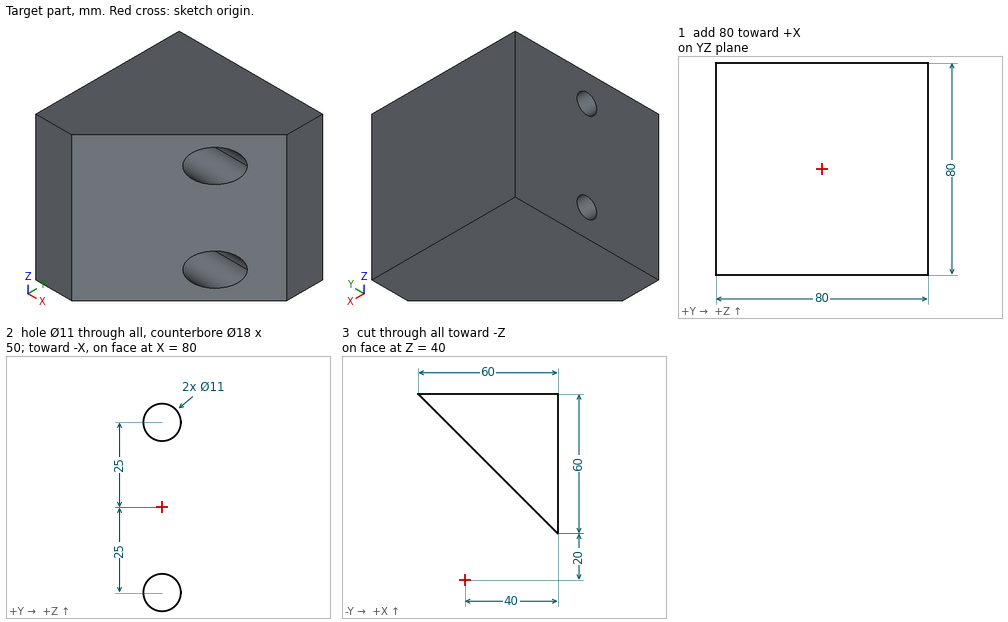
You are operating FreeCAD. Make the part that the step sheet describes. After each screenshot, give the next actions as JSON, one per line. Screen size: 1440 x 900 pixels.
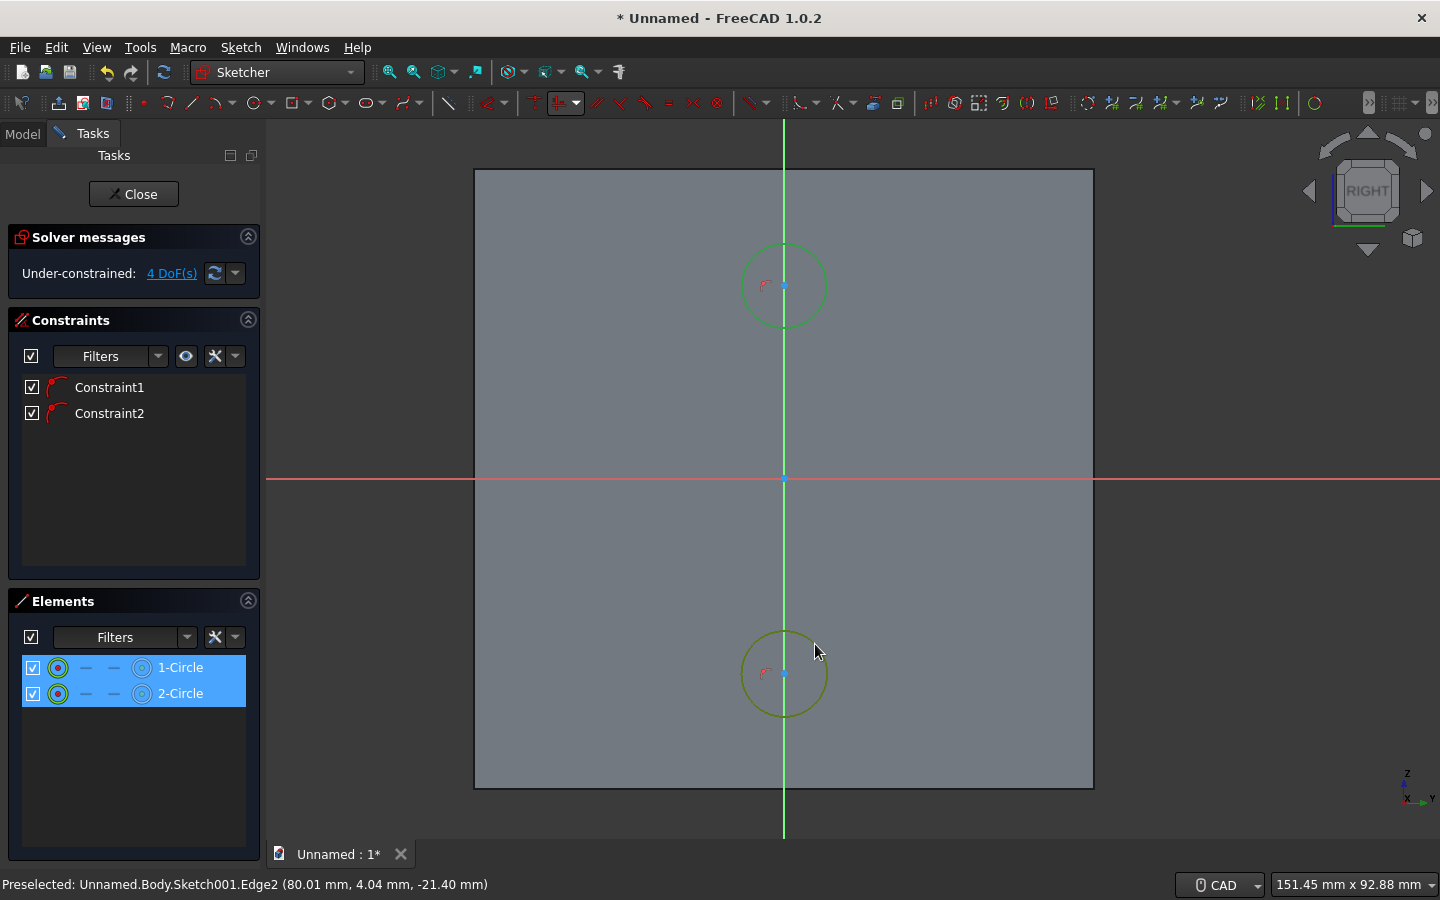
{"action": "key", "text": "e"}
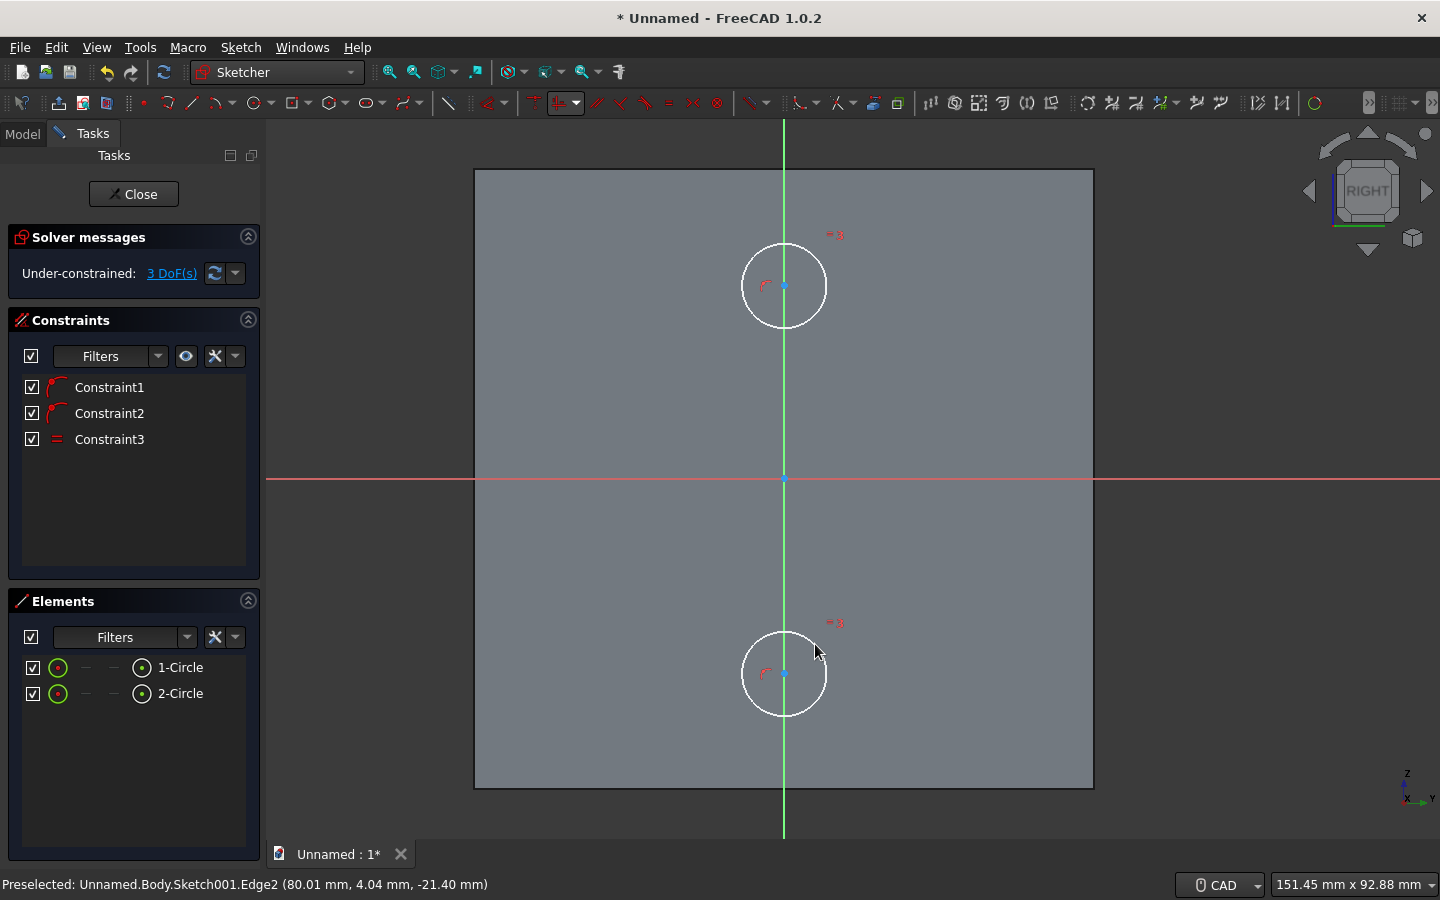
{"action": "key", "text": "d"}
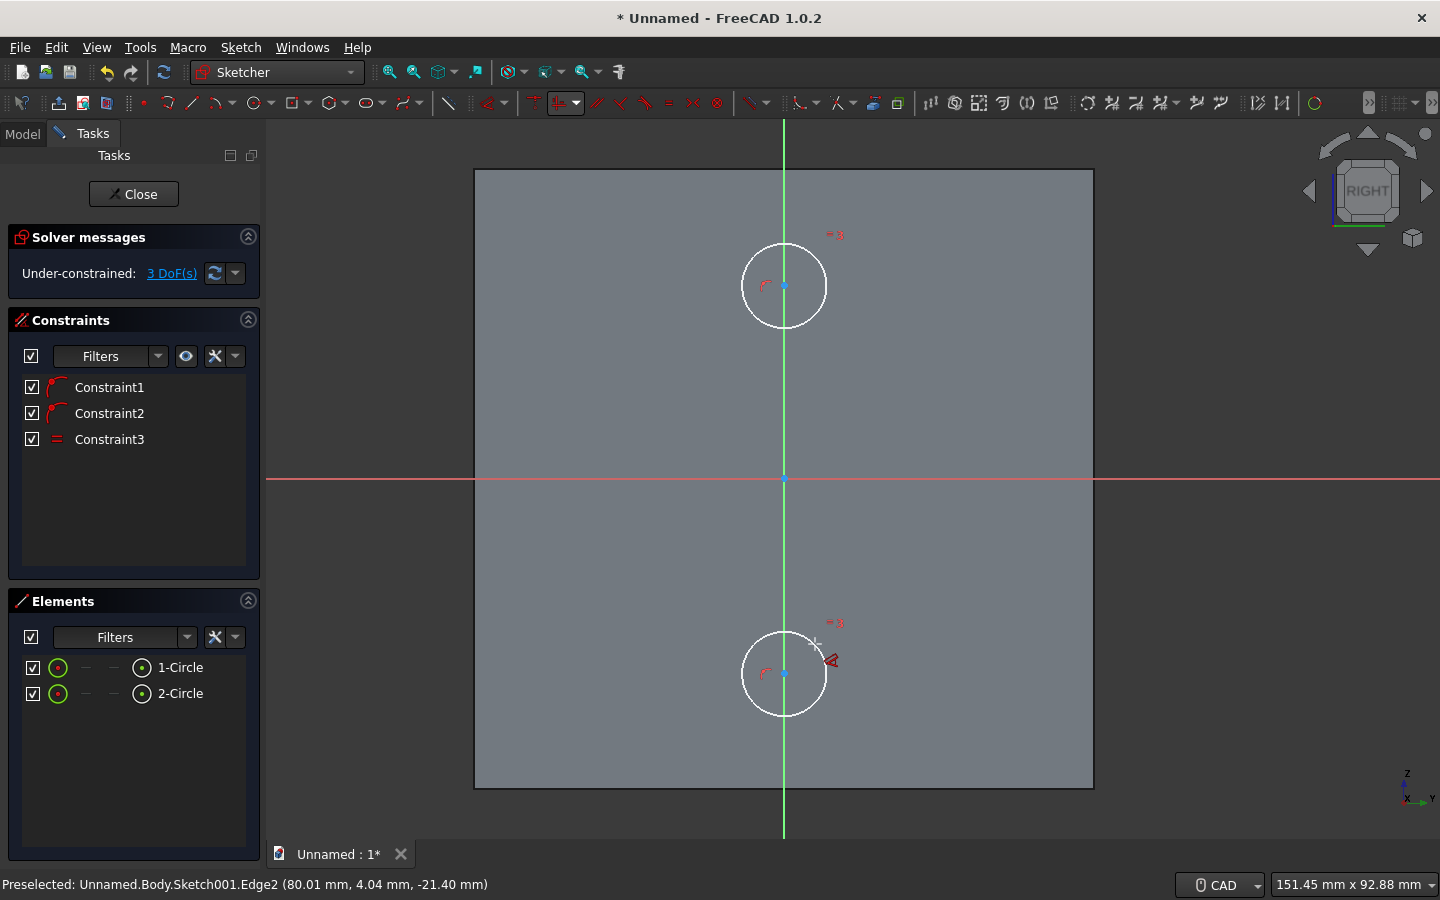
{"action": "left_click", "coordinate": [814, 256]}
{"action": "left_click", "coordinate": [837, 233]}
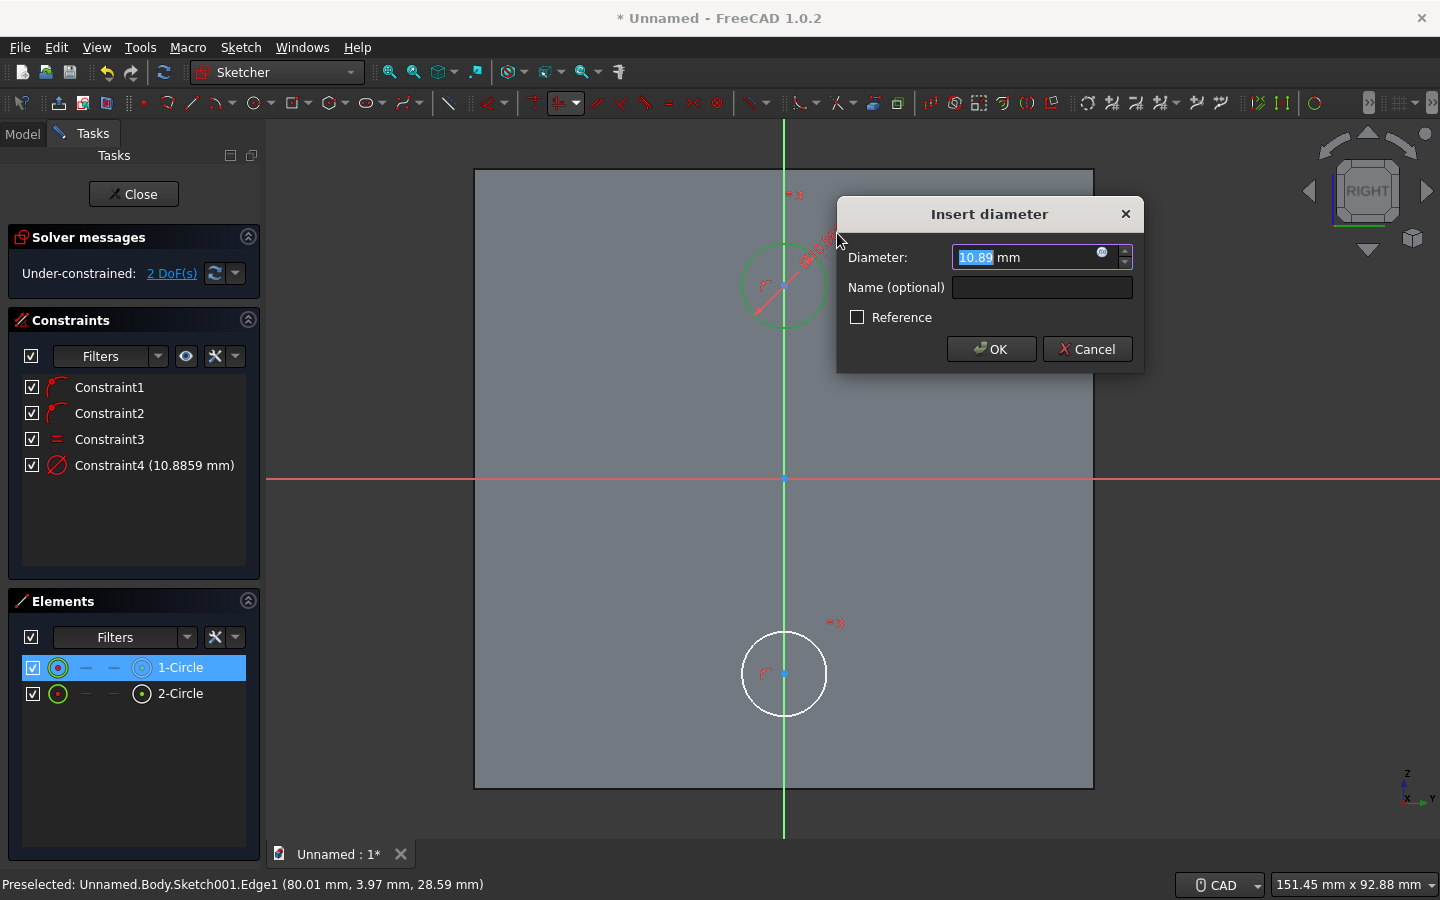
{"action": "type", "text": "11"}
{"action": "key", "text": "Return"}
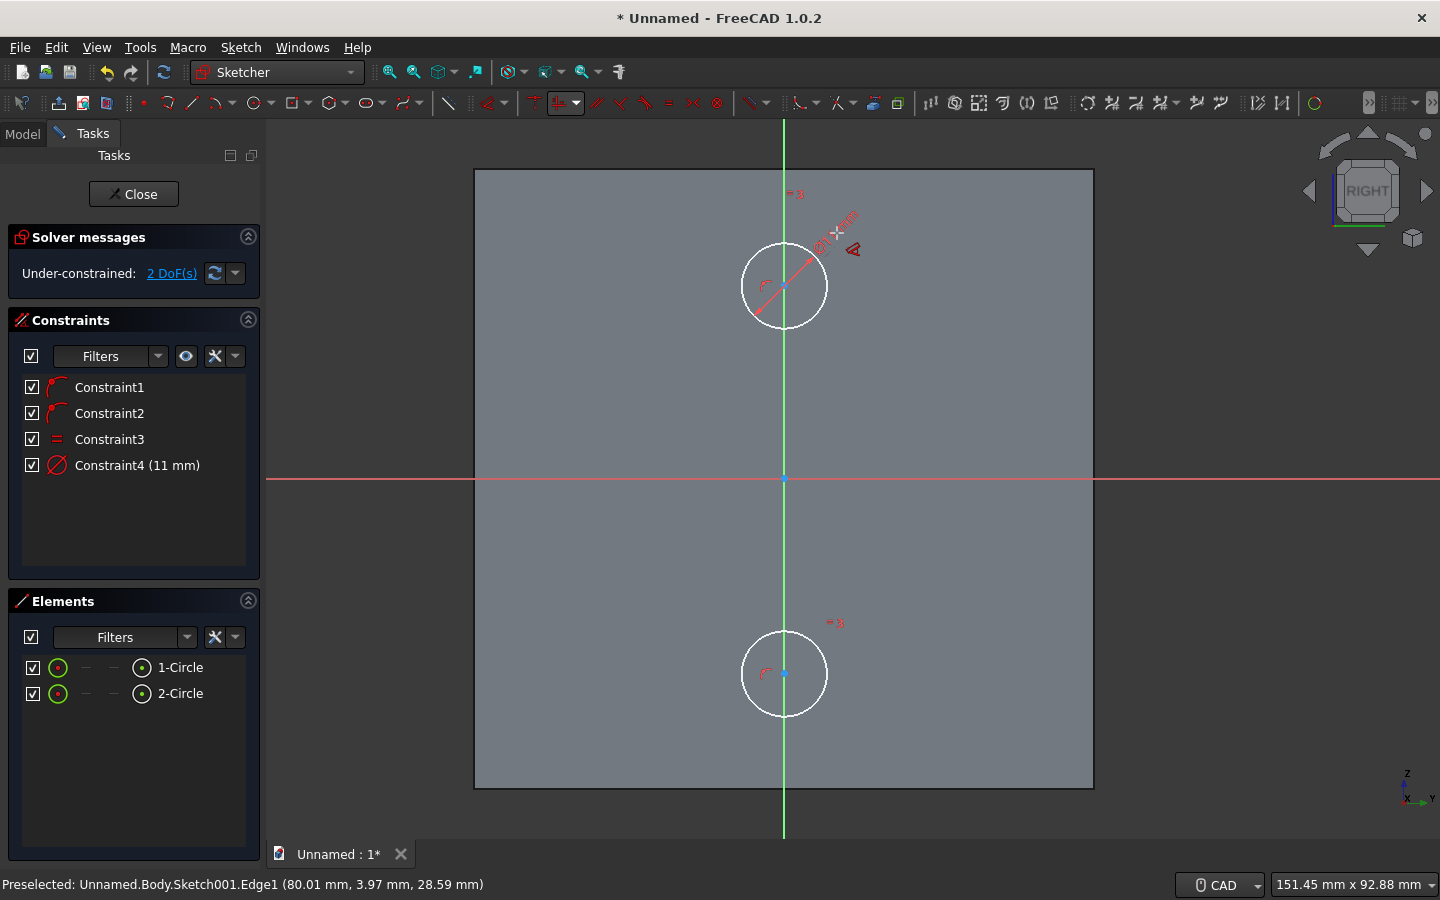
{"action": "left_click", "coordinate": [784, 286]}
{"action": "left_click", "coordinate": [818, 382]}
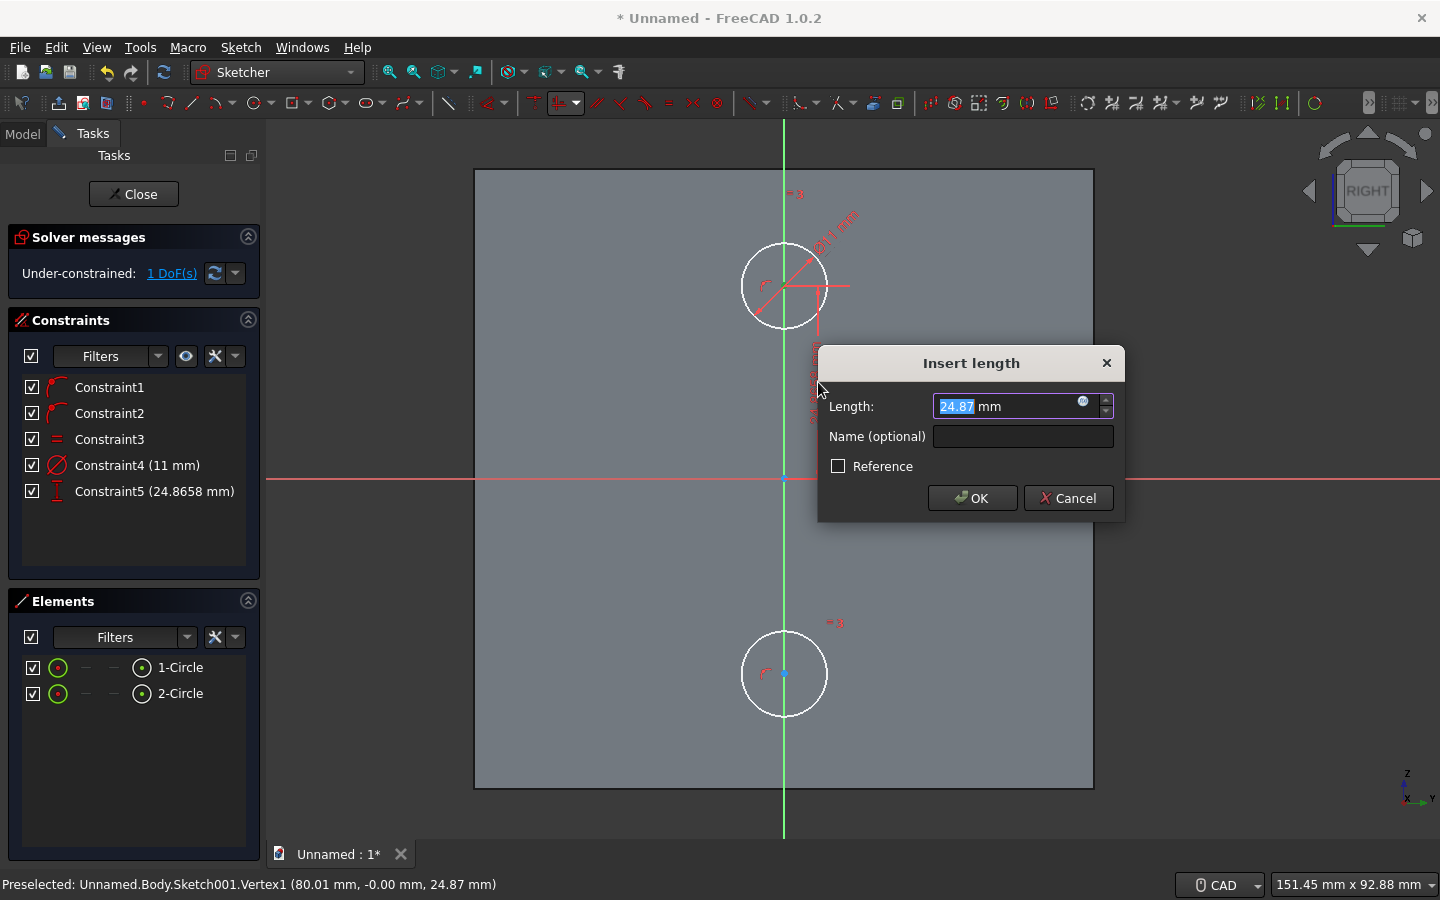
{"action": "type", "text": "25"}
{"action": "key", "text": "Return"}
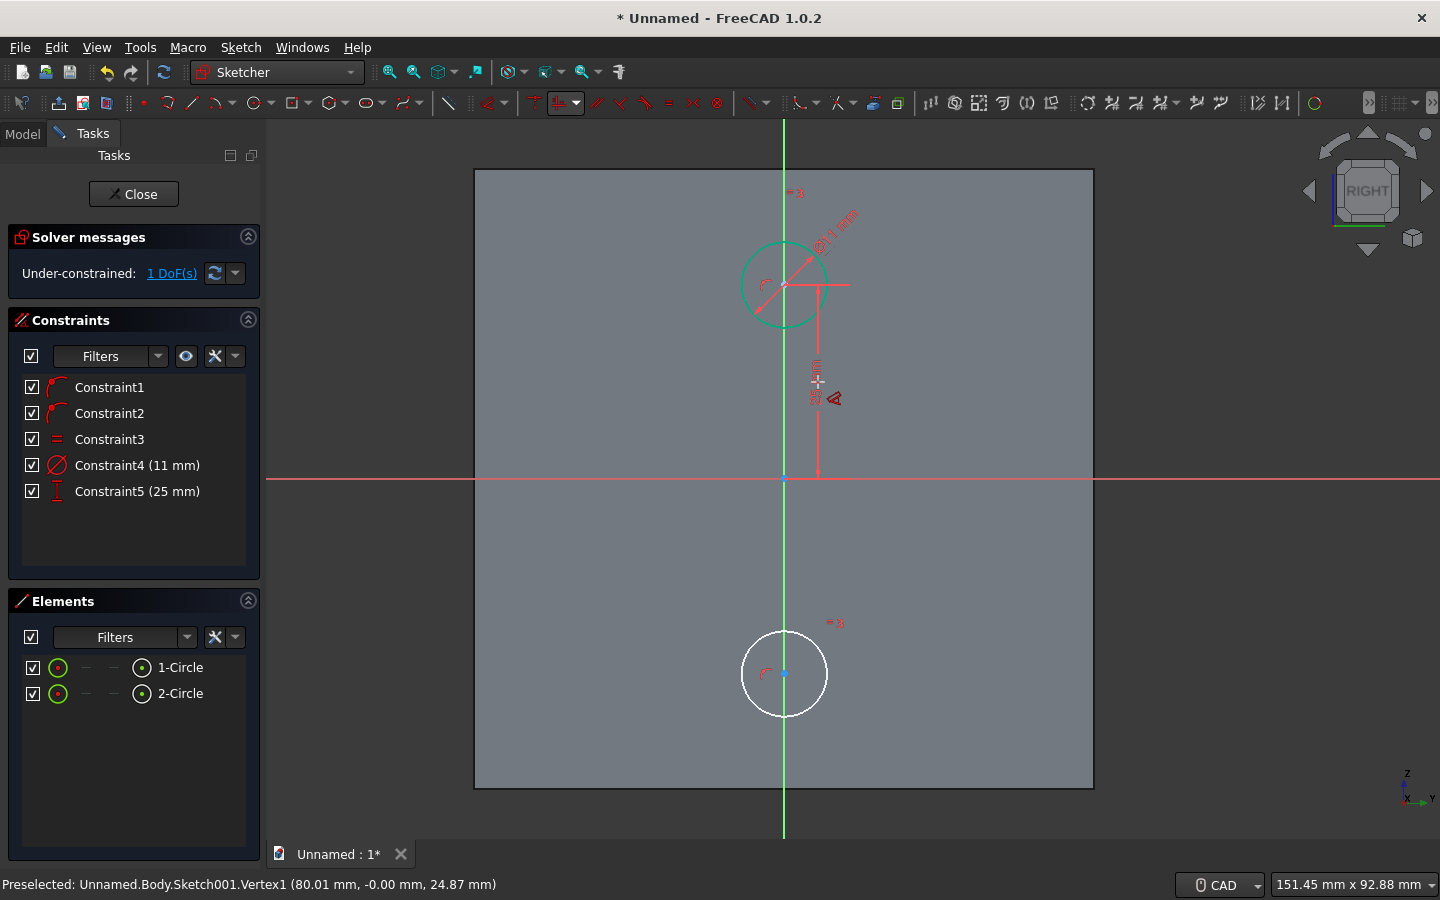
{"action": "left_click", "coordinate": [784, 674]}
{"action": "left_click", "coordinate": [818, 576]}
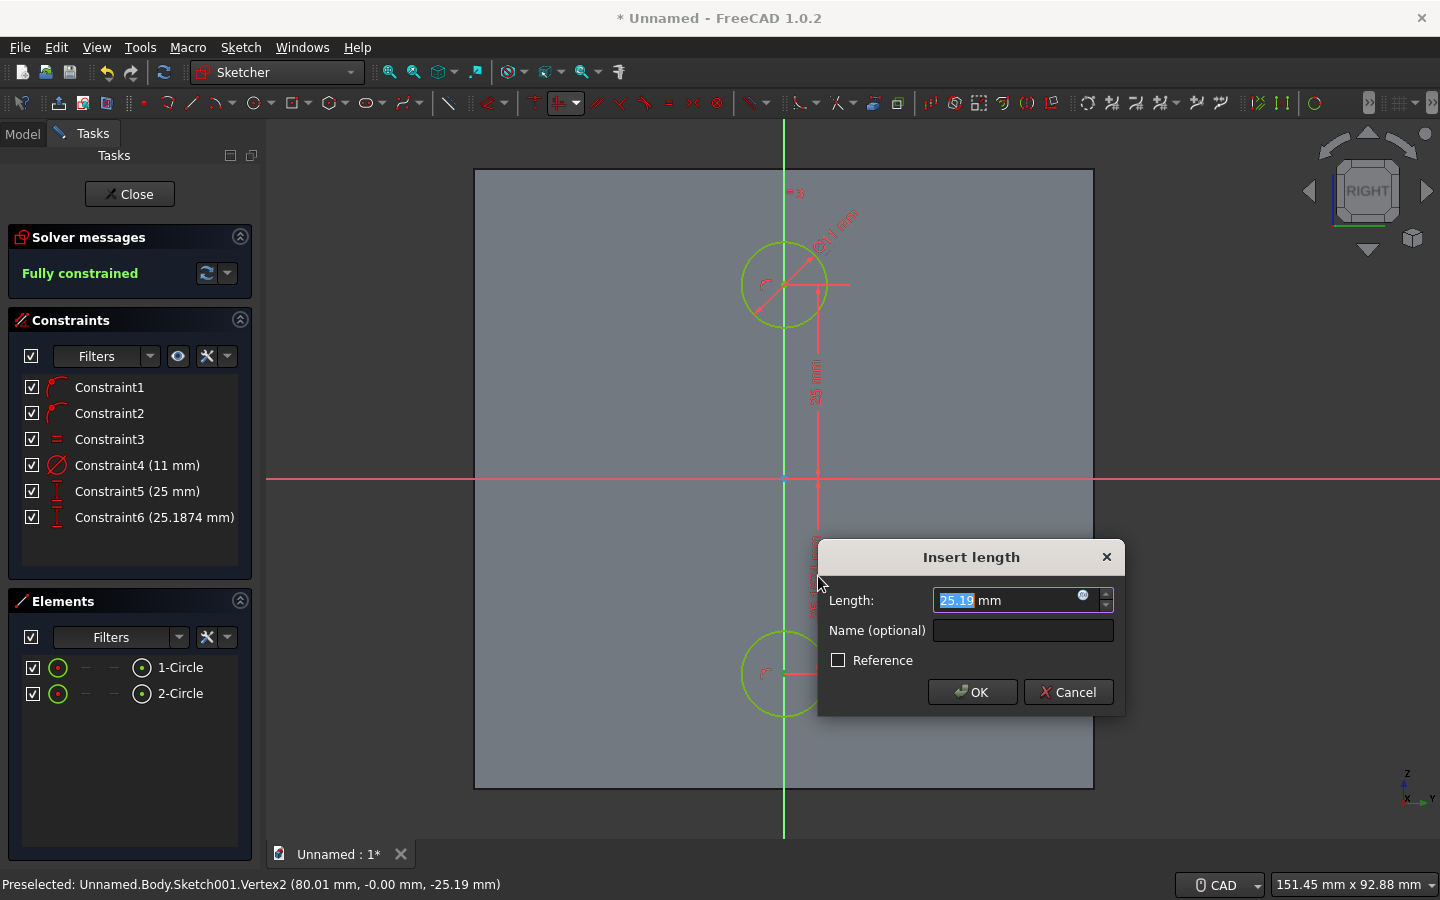
{"action": "type", "text": "25"}
{"action": "key", "text": "Return"}
{"action": "key", "text": "Escape"}